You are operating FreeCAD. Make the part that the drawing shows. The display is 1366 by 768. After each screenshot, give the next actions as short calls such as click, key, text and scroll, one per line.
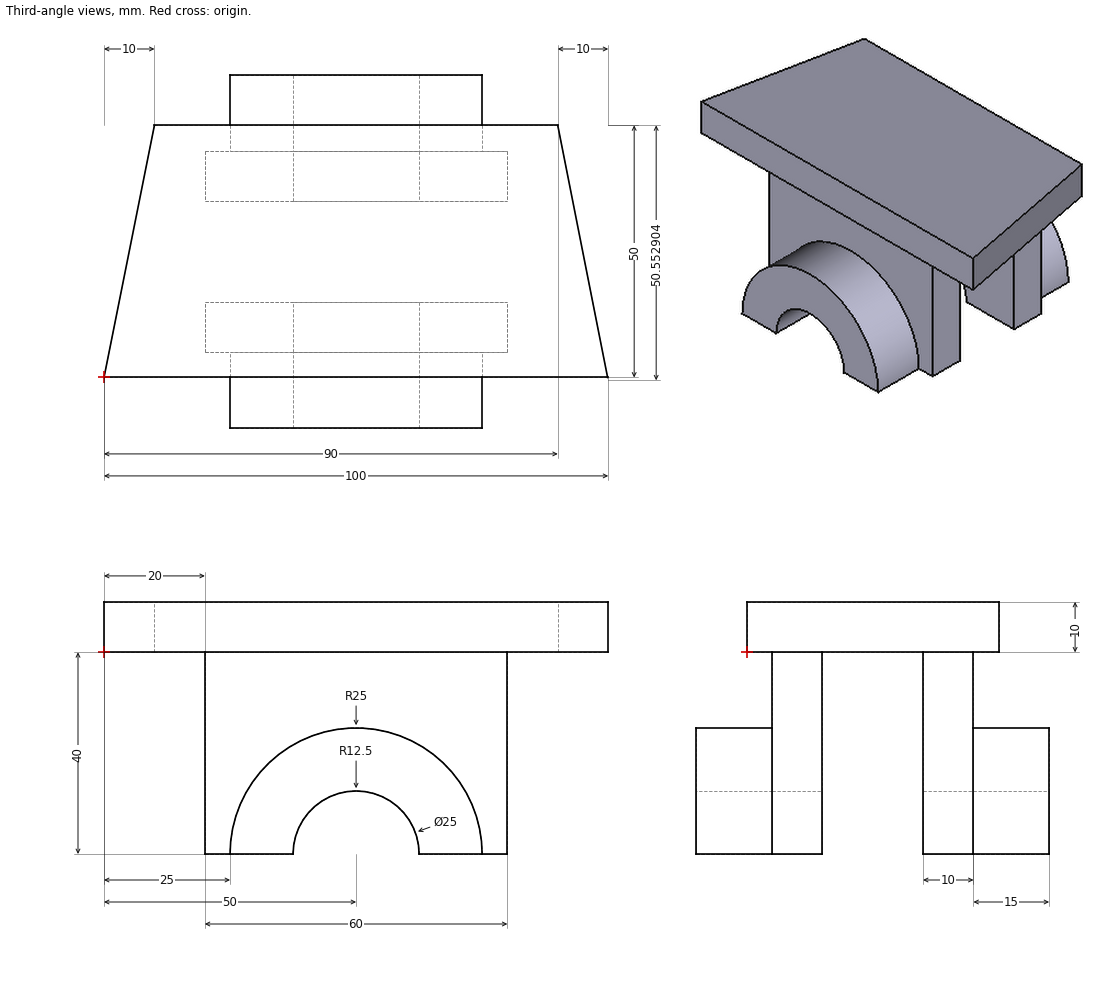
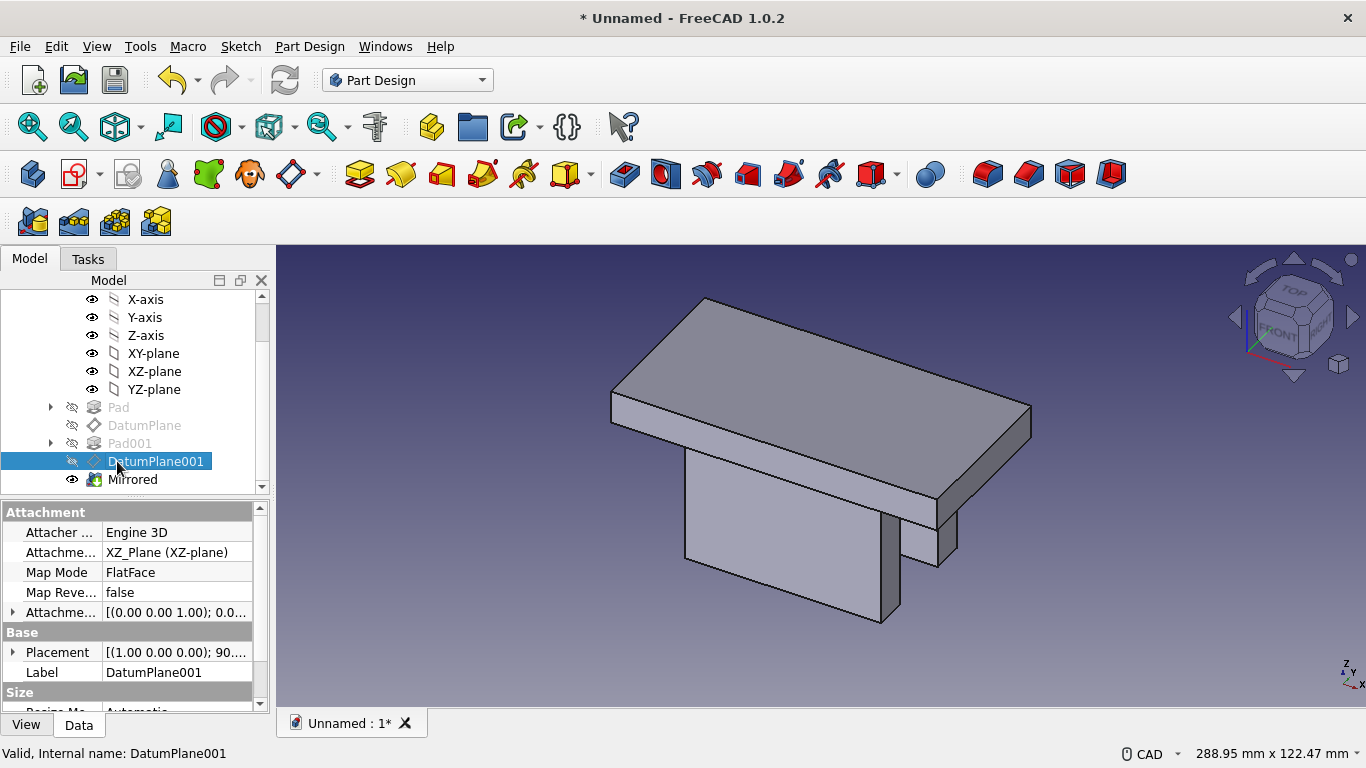
key(4)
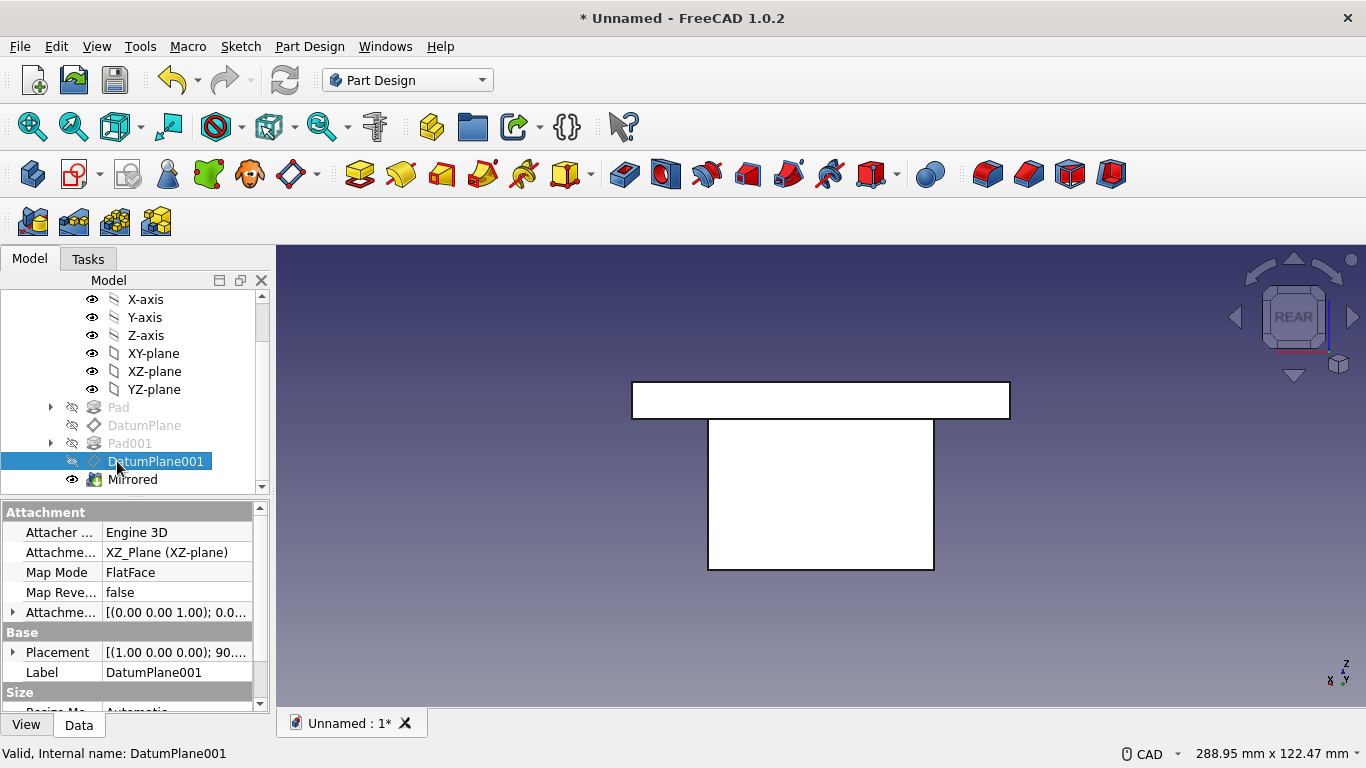
key(v)
key(f)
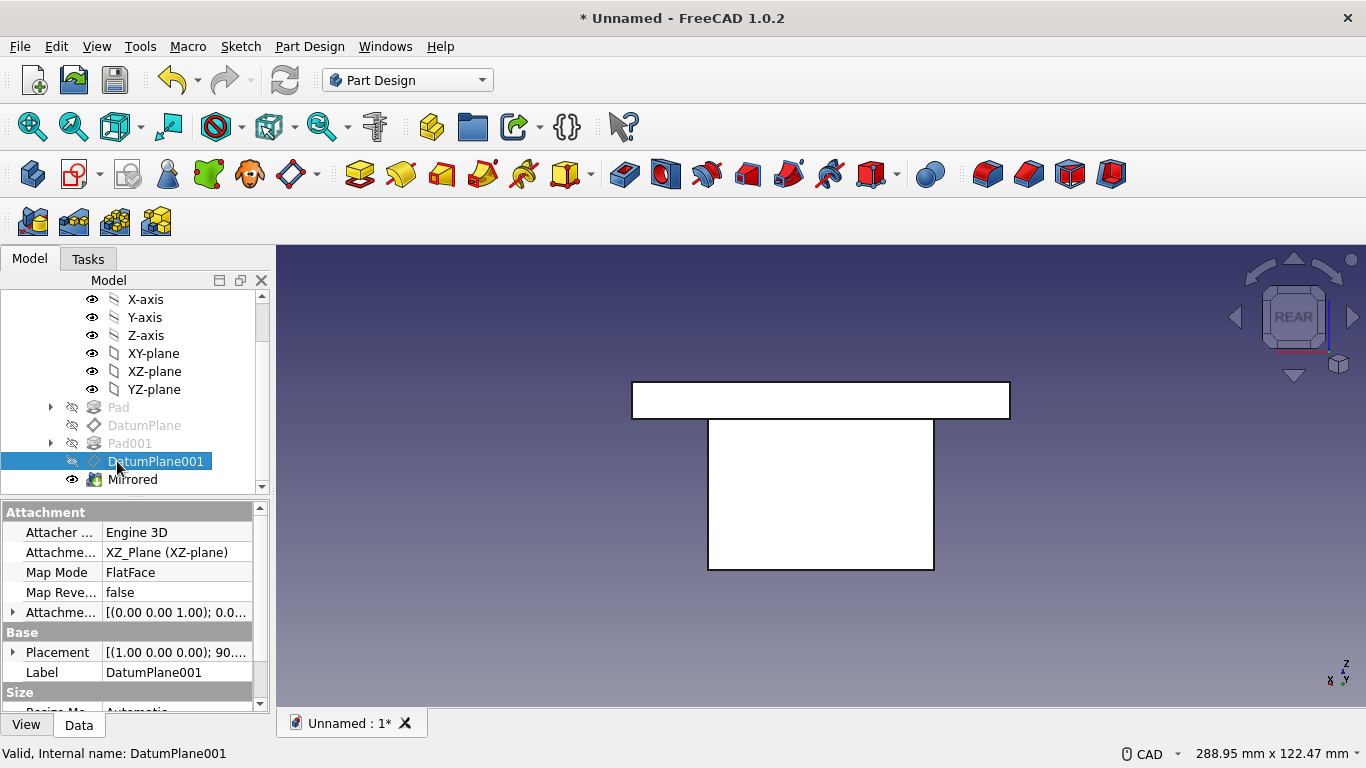
click(789, 494)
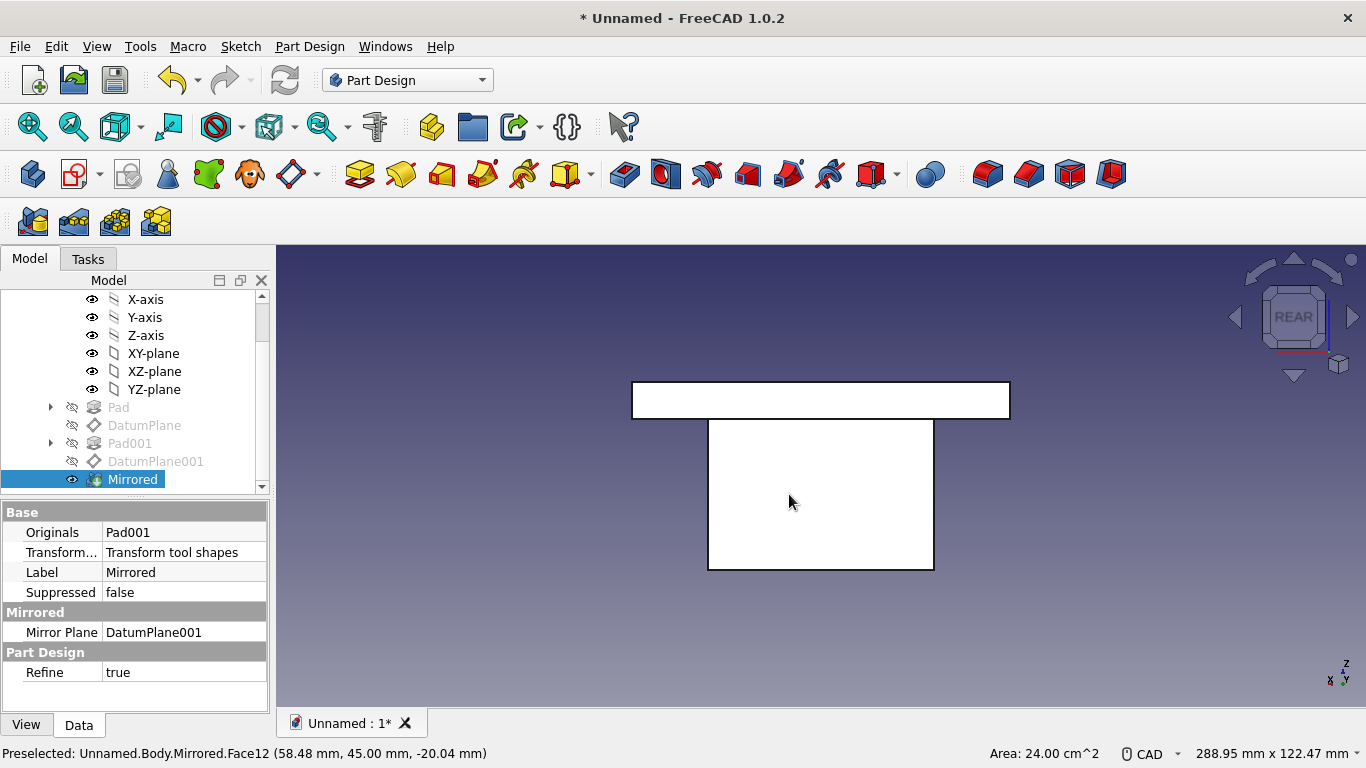
click(74, 174)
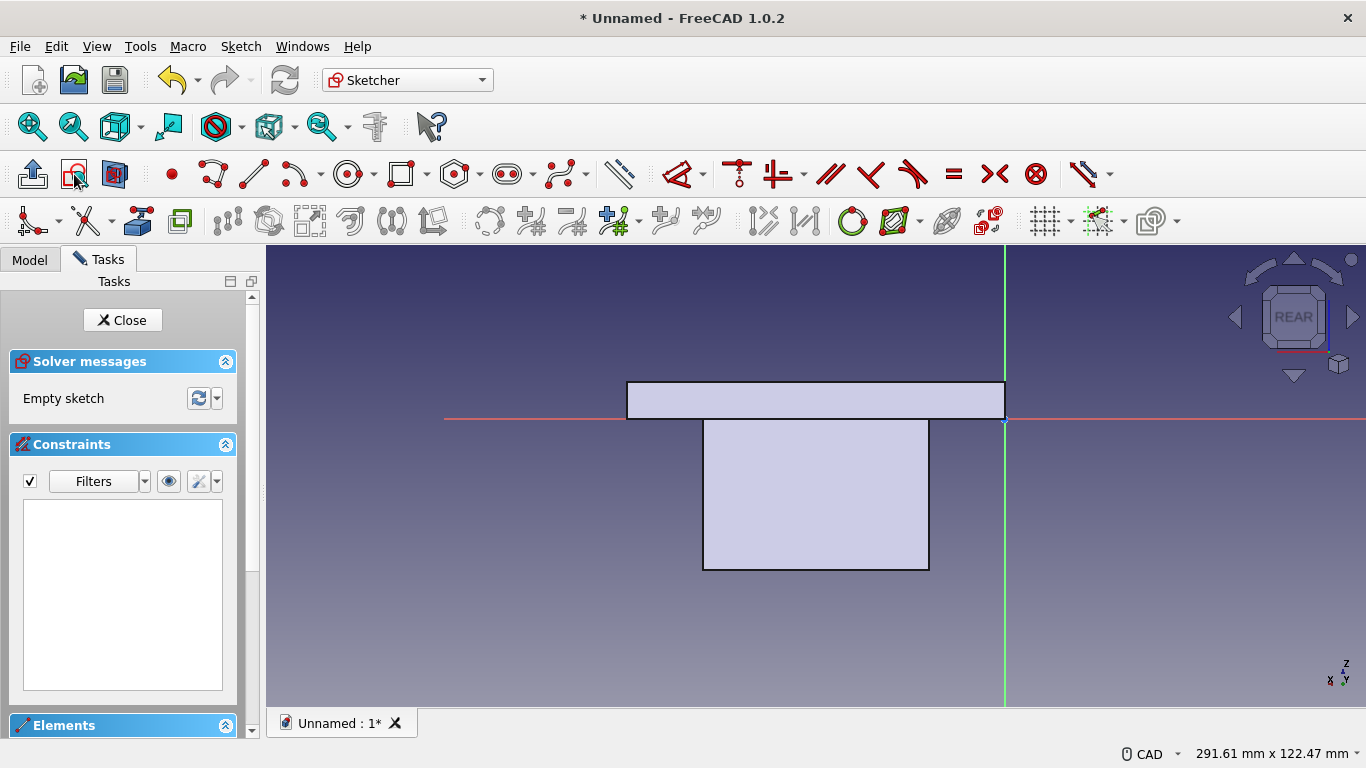
key(q)
key(s)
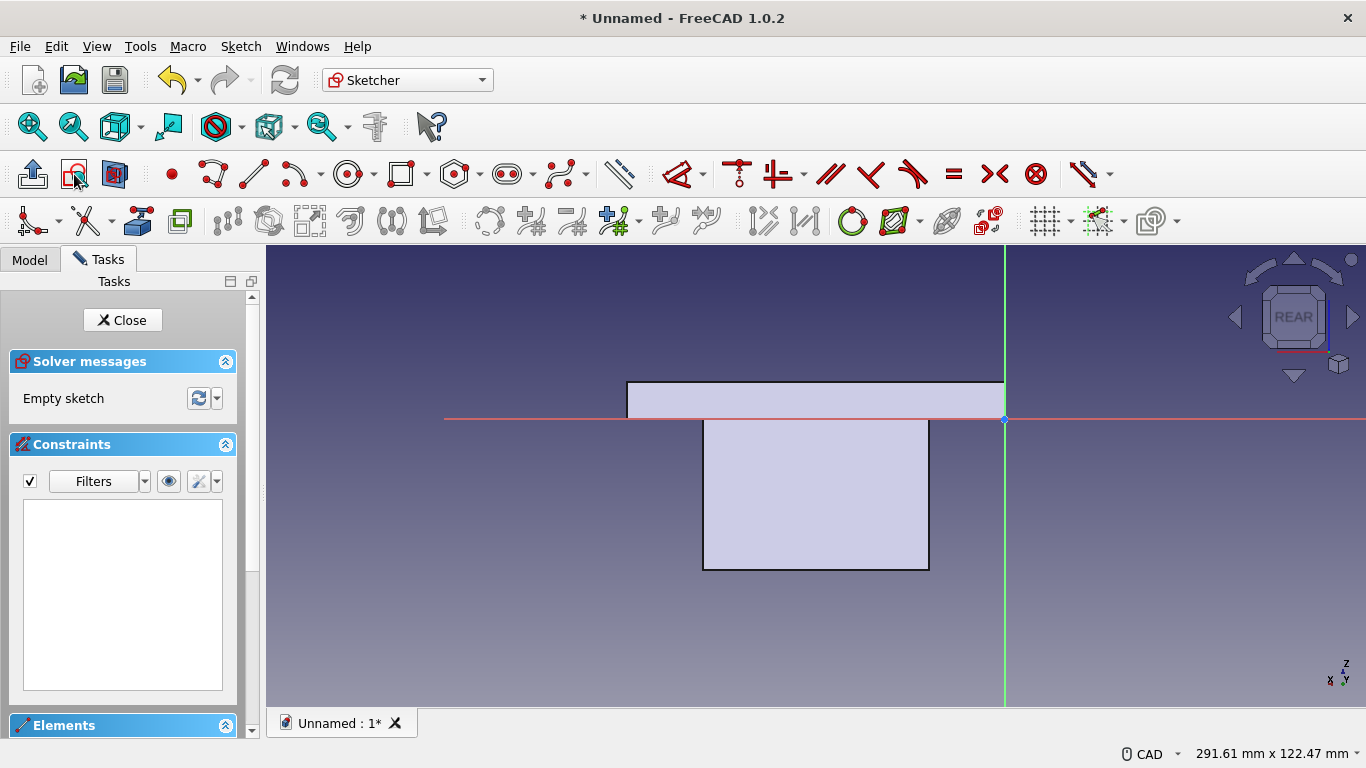
scroll(846, 611, up, 6)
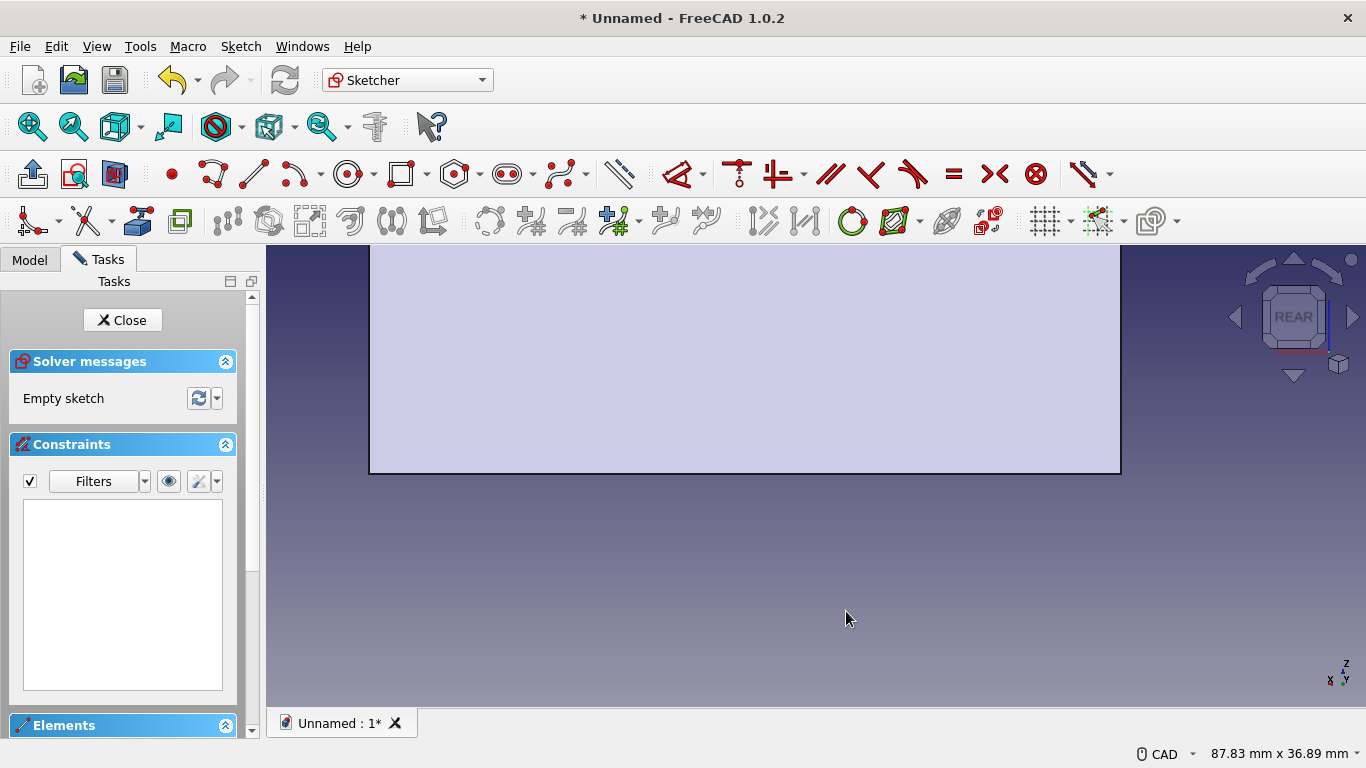
key(g)
key(c)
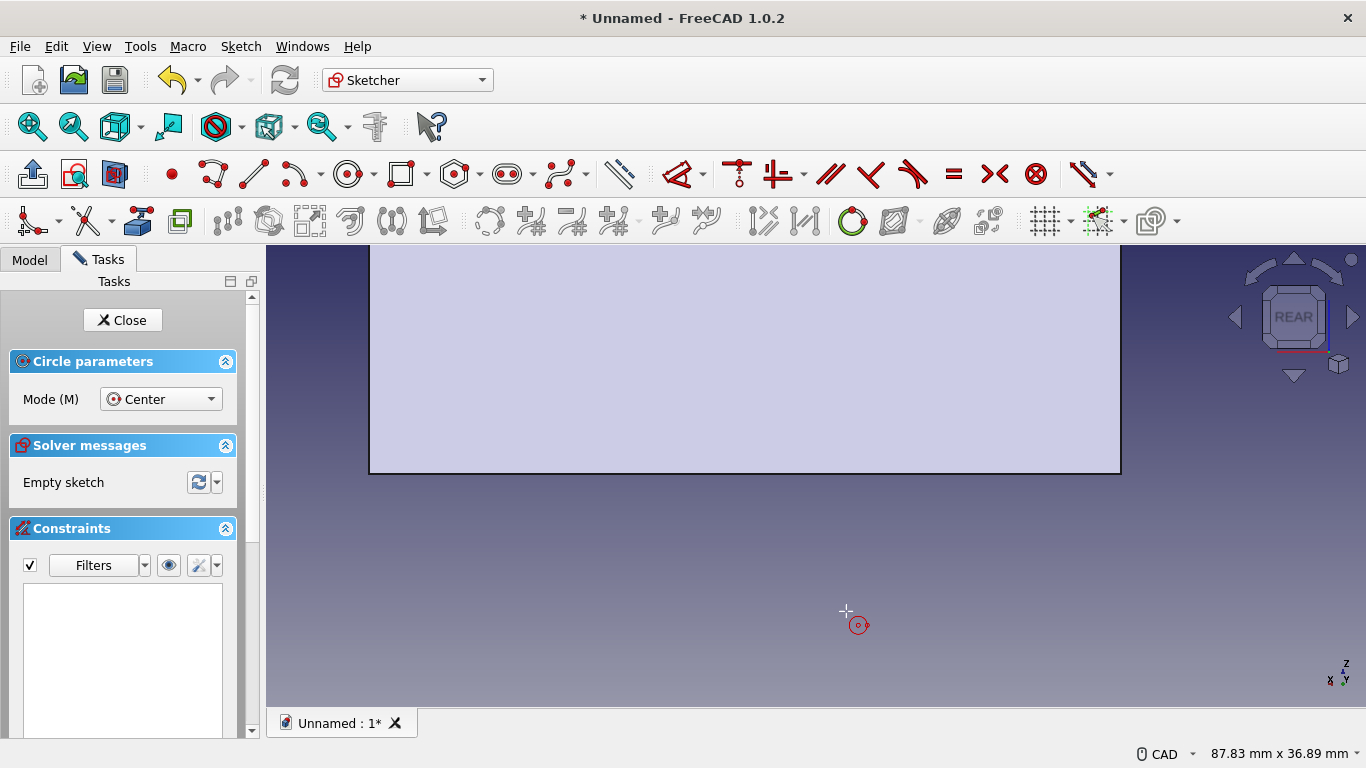
click(745, 474)
click(856, 363)
key(Escape)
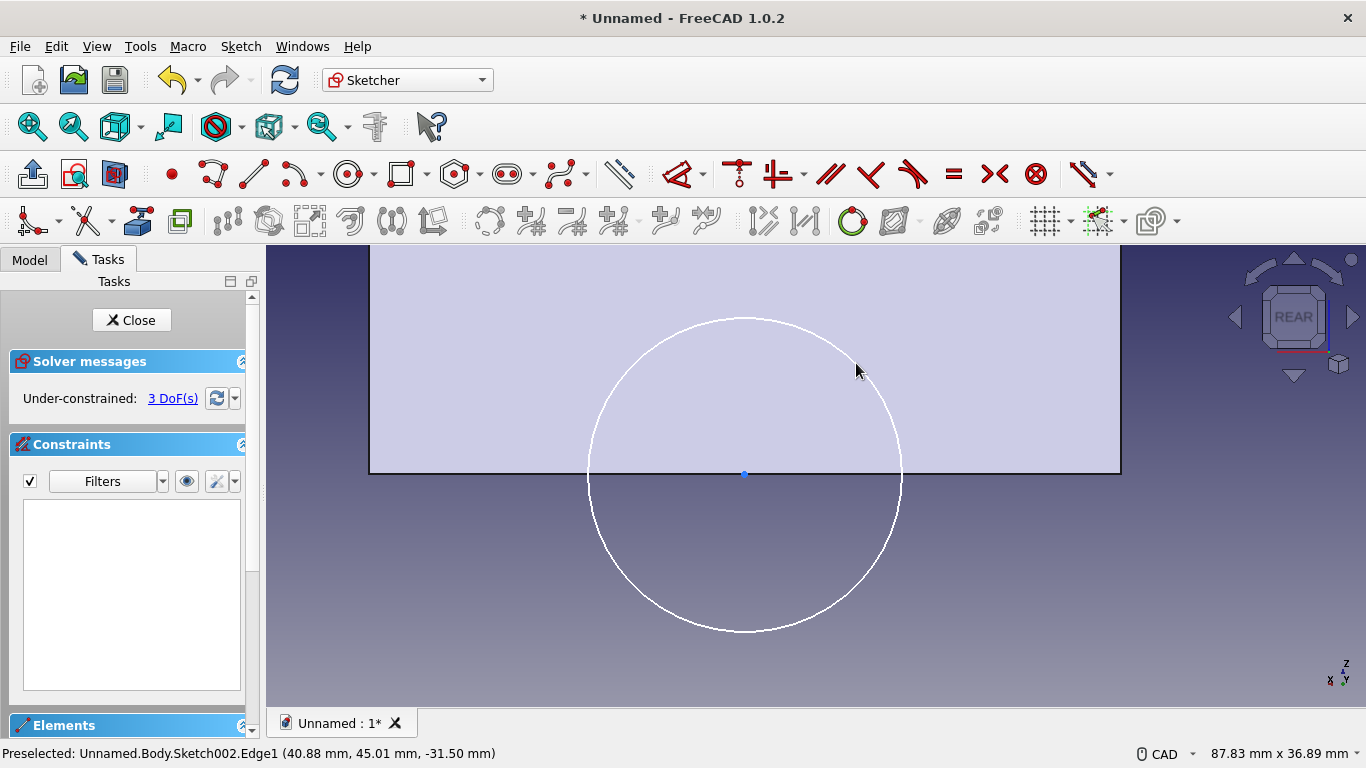
key(d)